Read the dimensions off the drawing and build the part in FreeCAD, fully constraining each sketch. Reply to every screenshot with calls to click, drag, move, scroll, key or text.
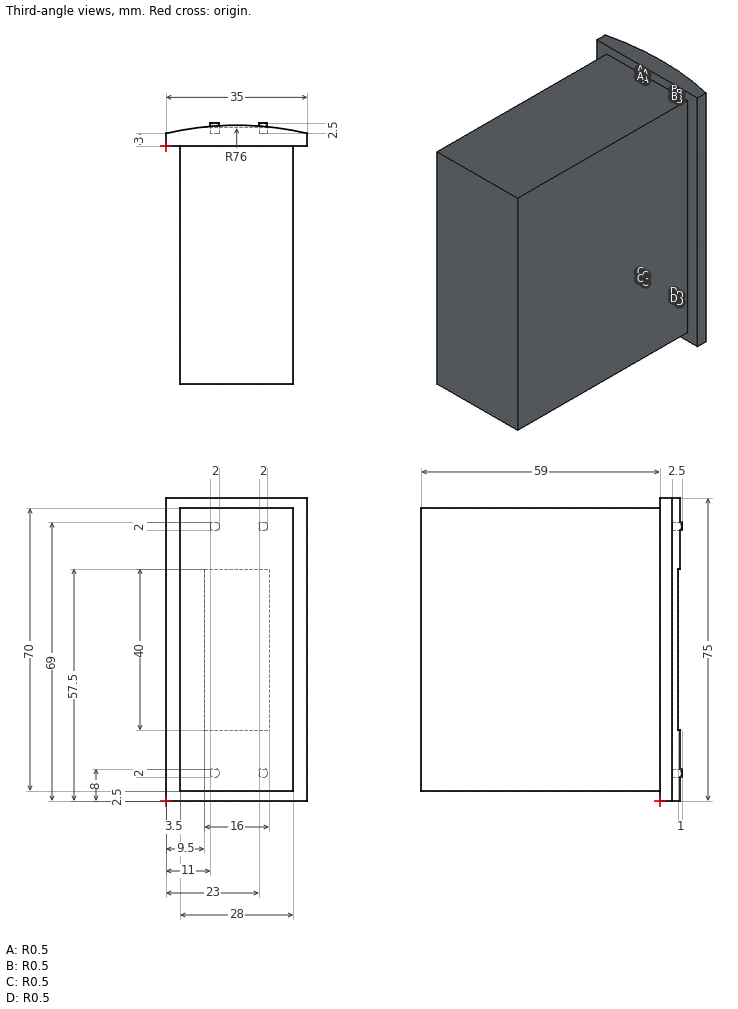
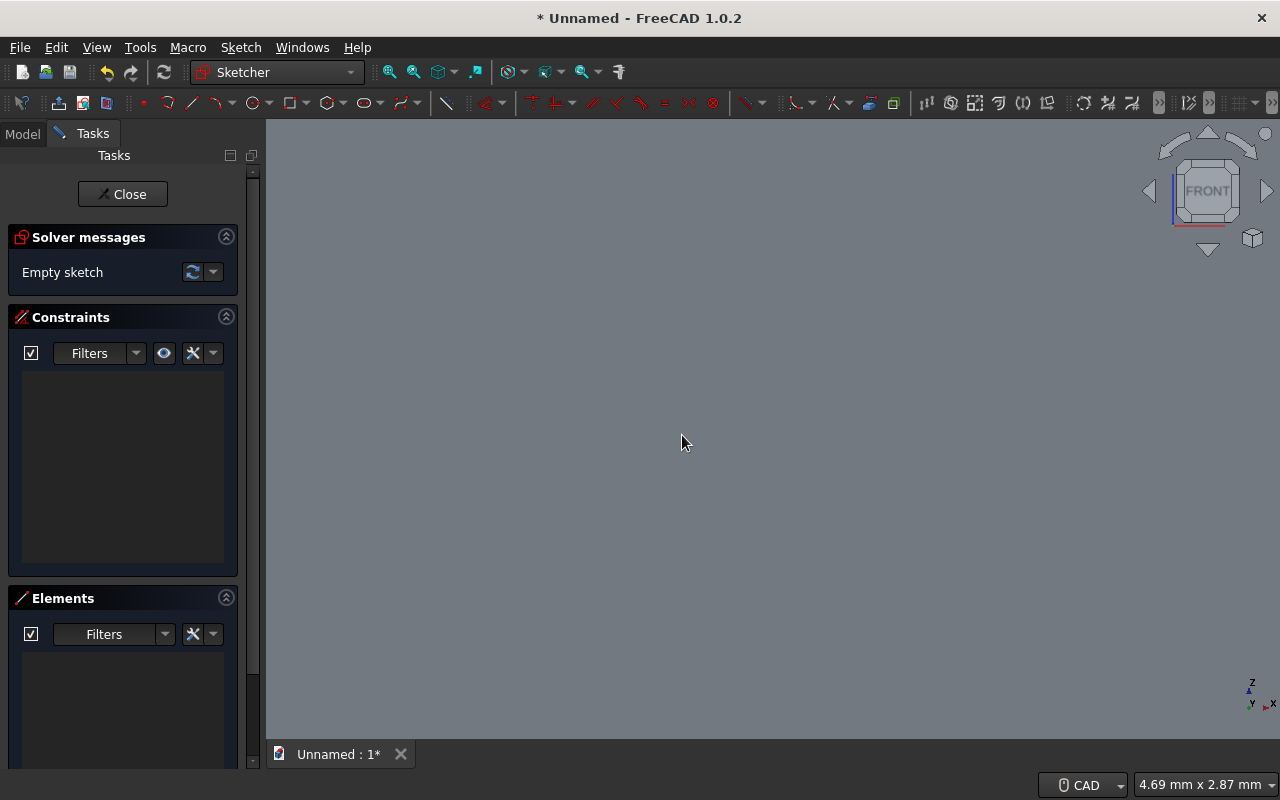
key(g)
key(r)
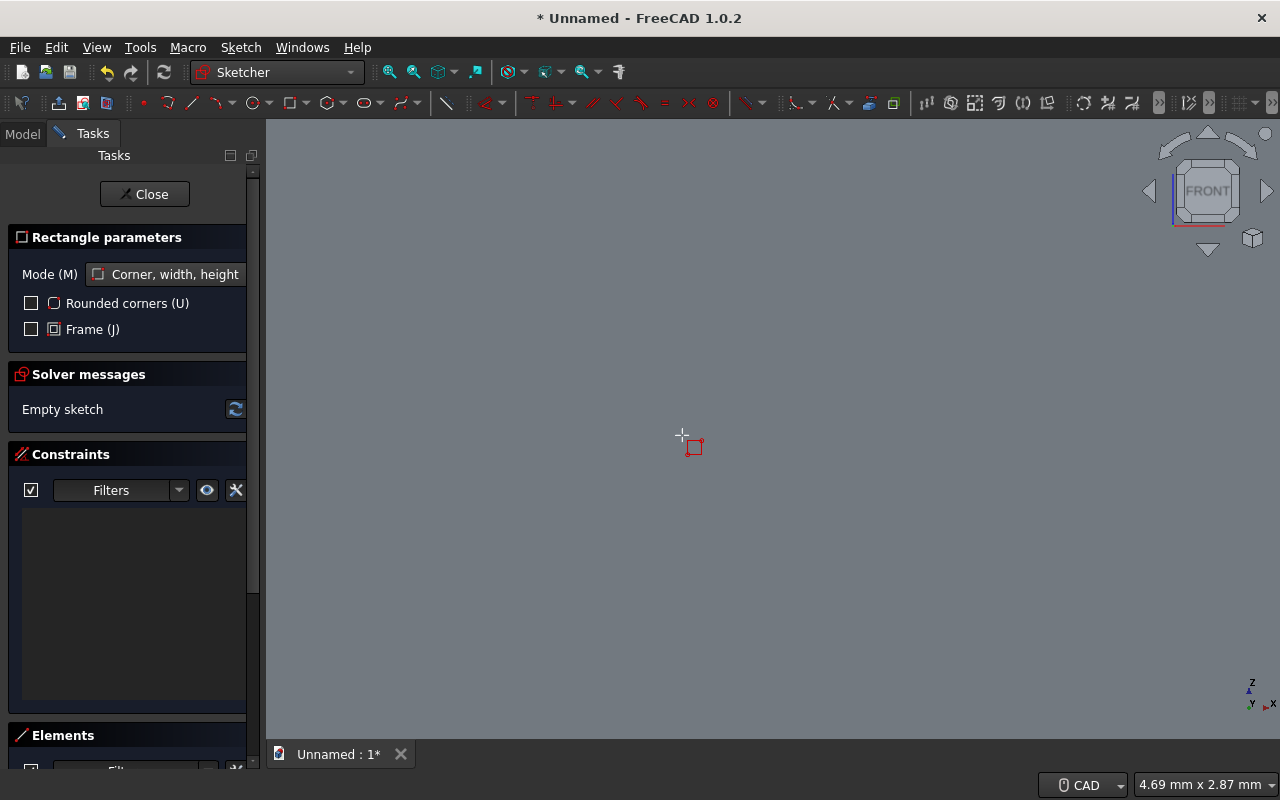
click(488, 213)
click(920, 645)
key(Escape)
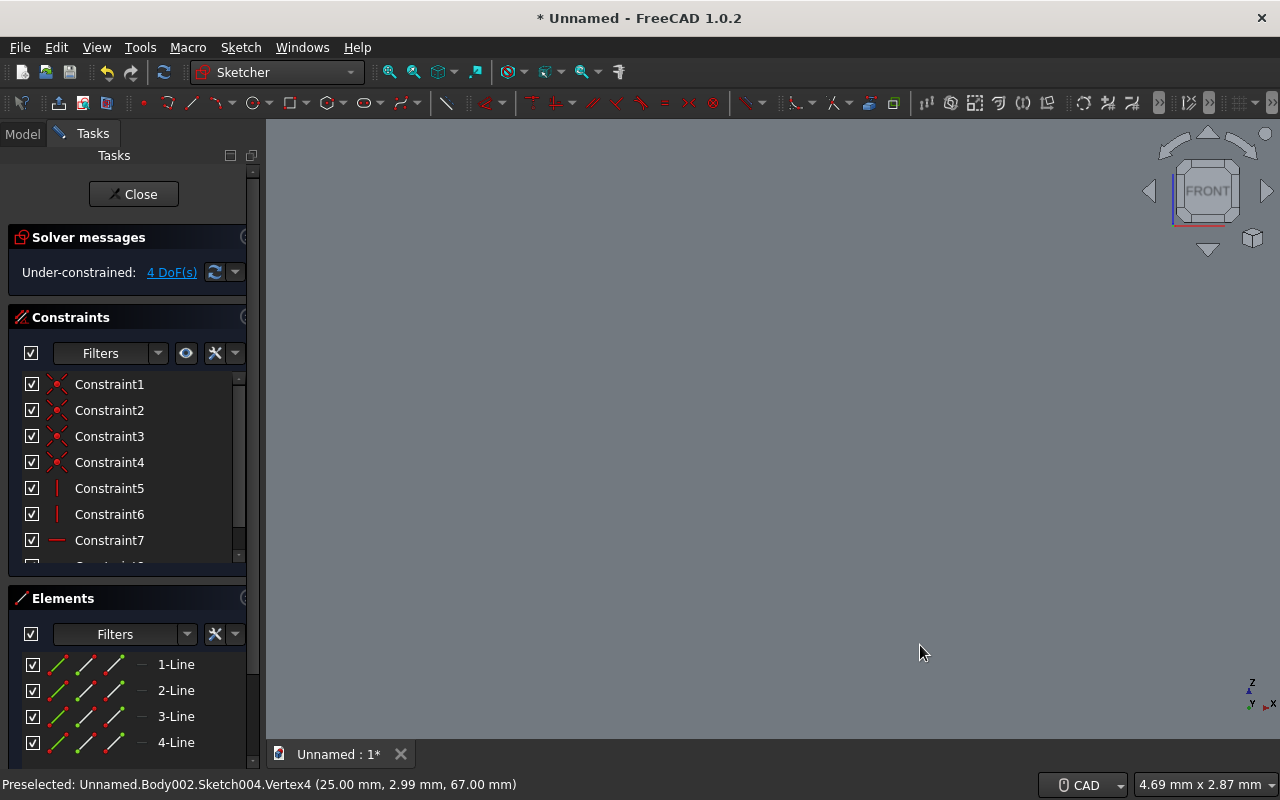
click(486, 104)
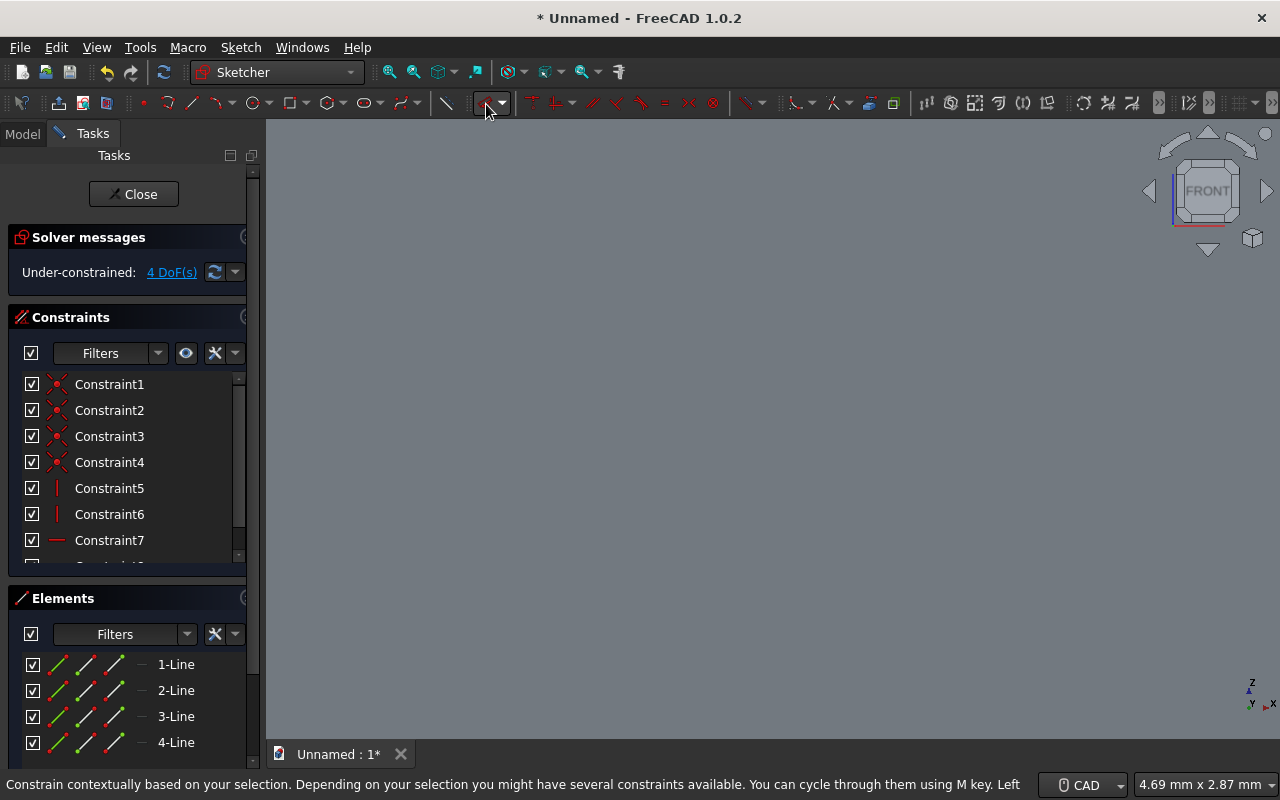
click(488, 344)
click(454, 430)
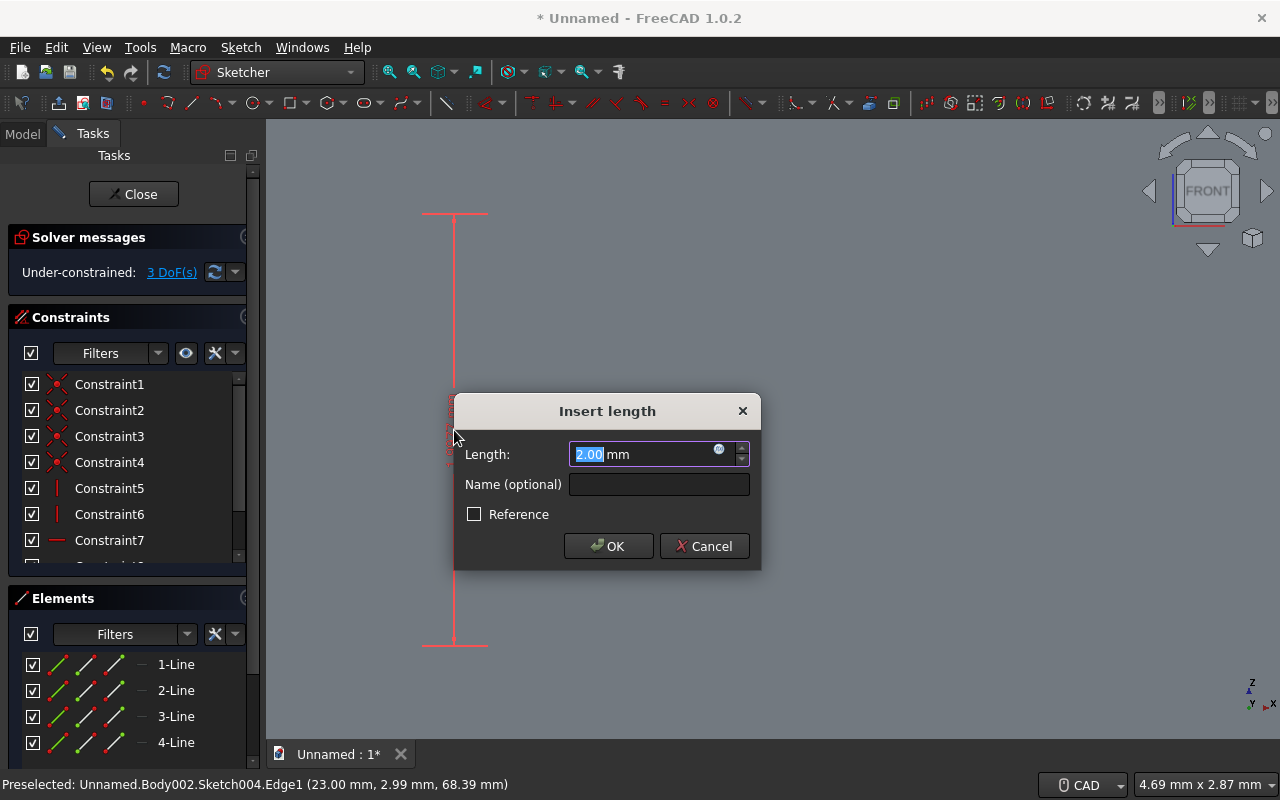
text(2)
key(Return)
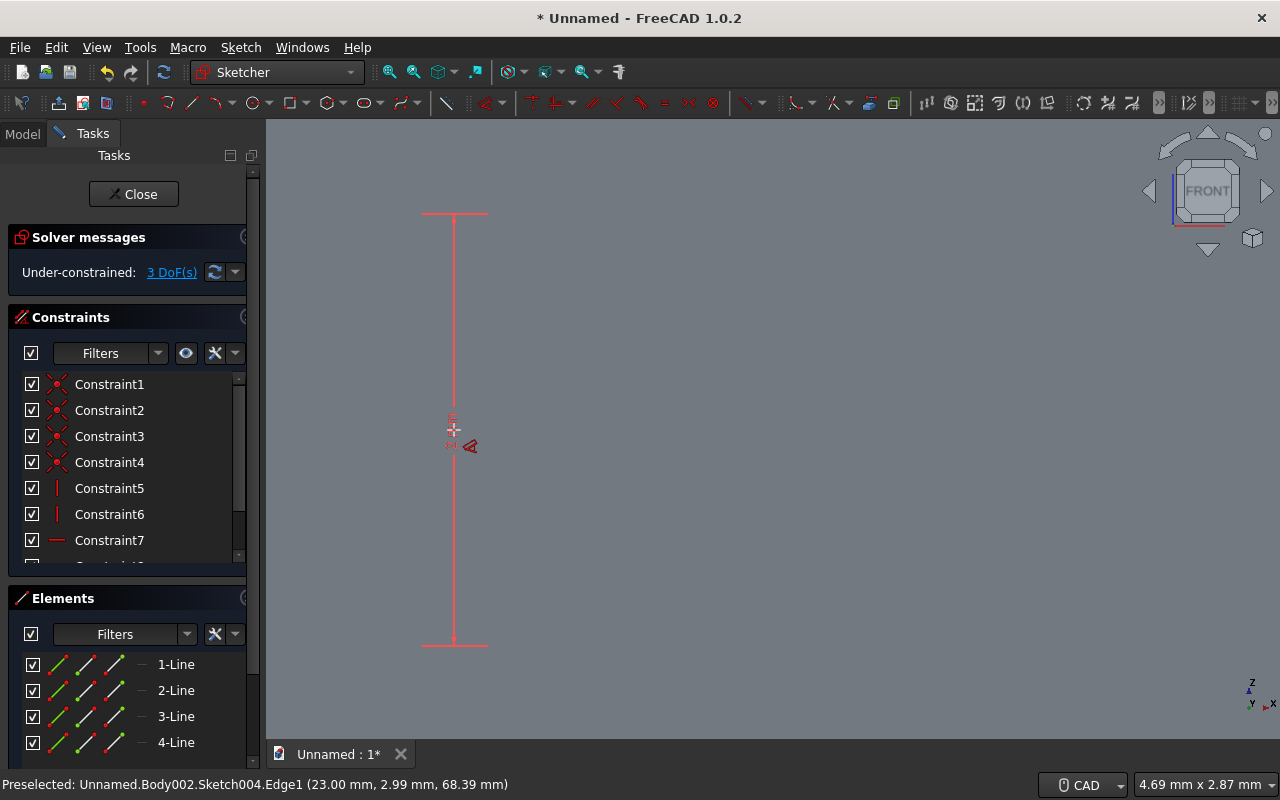
click(618, 646)
click(704, 680)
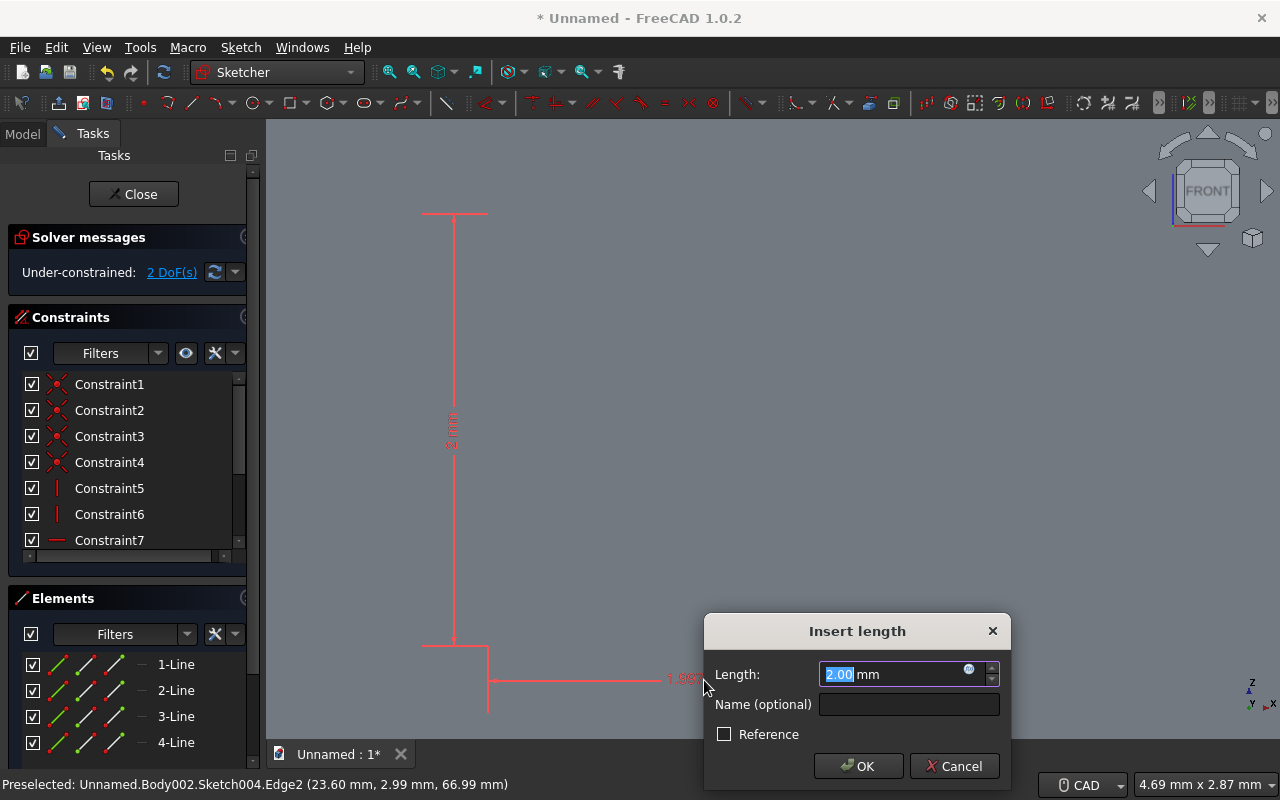
text(2)
key(Return)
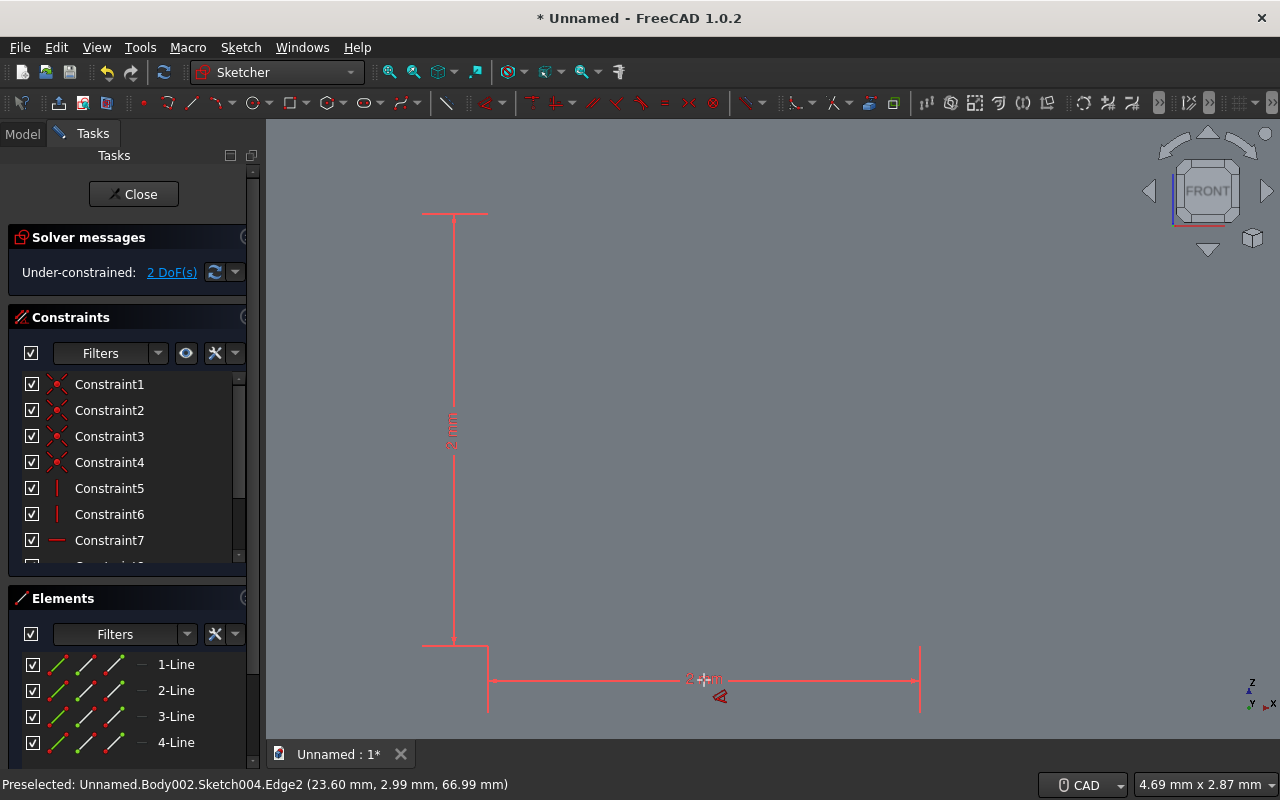
click(488, 214)
click(391, 180)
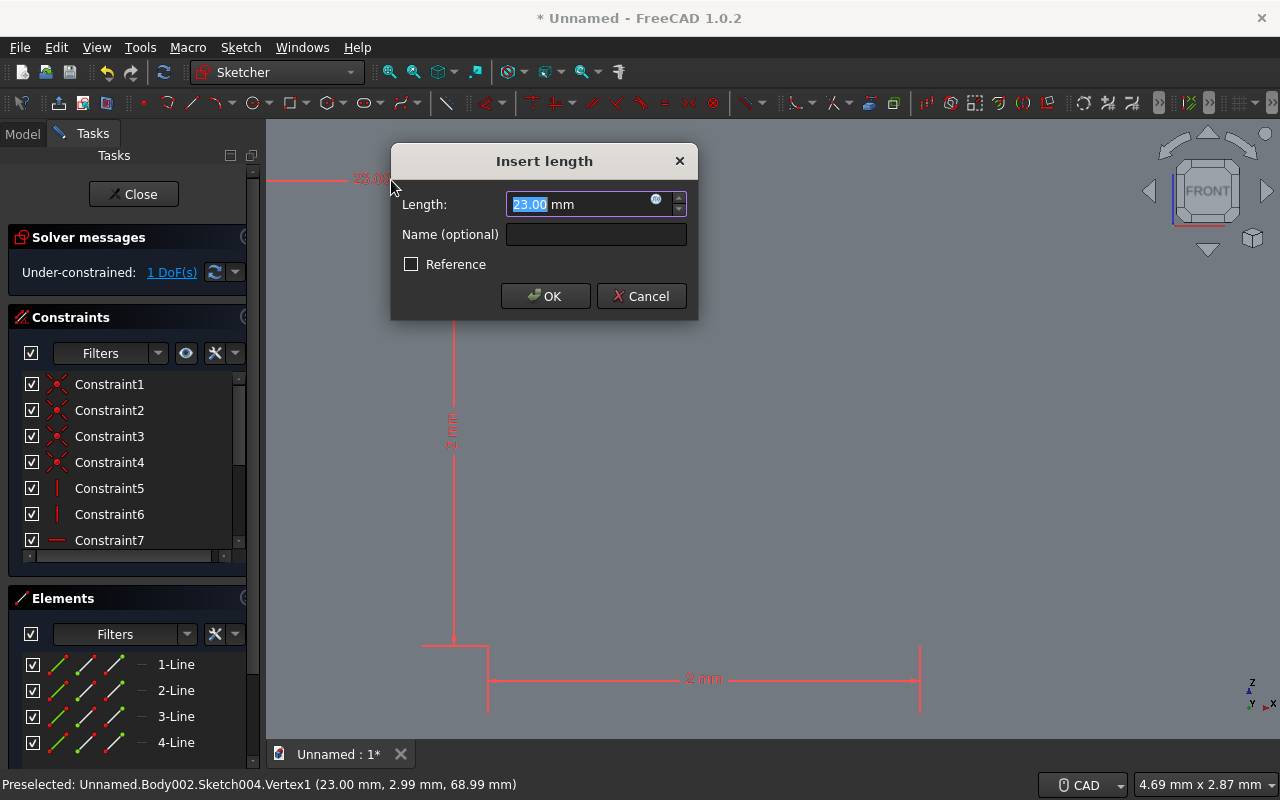
text(23)
key(Return)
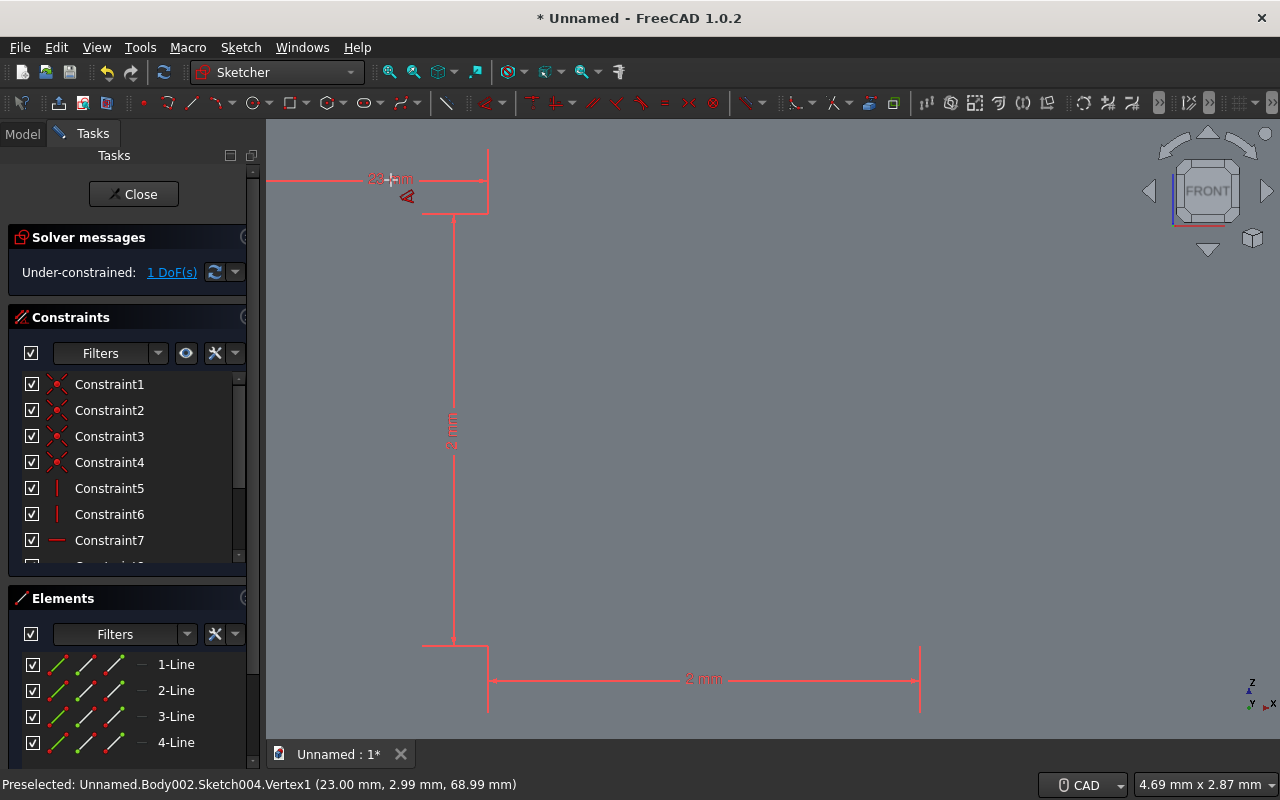
click(488, 214)
click(522, 463)